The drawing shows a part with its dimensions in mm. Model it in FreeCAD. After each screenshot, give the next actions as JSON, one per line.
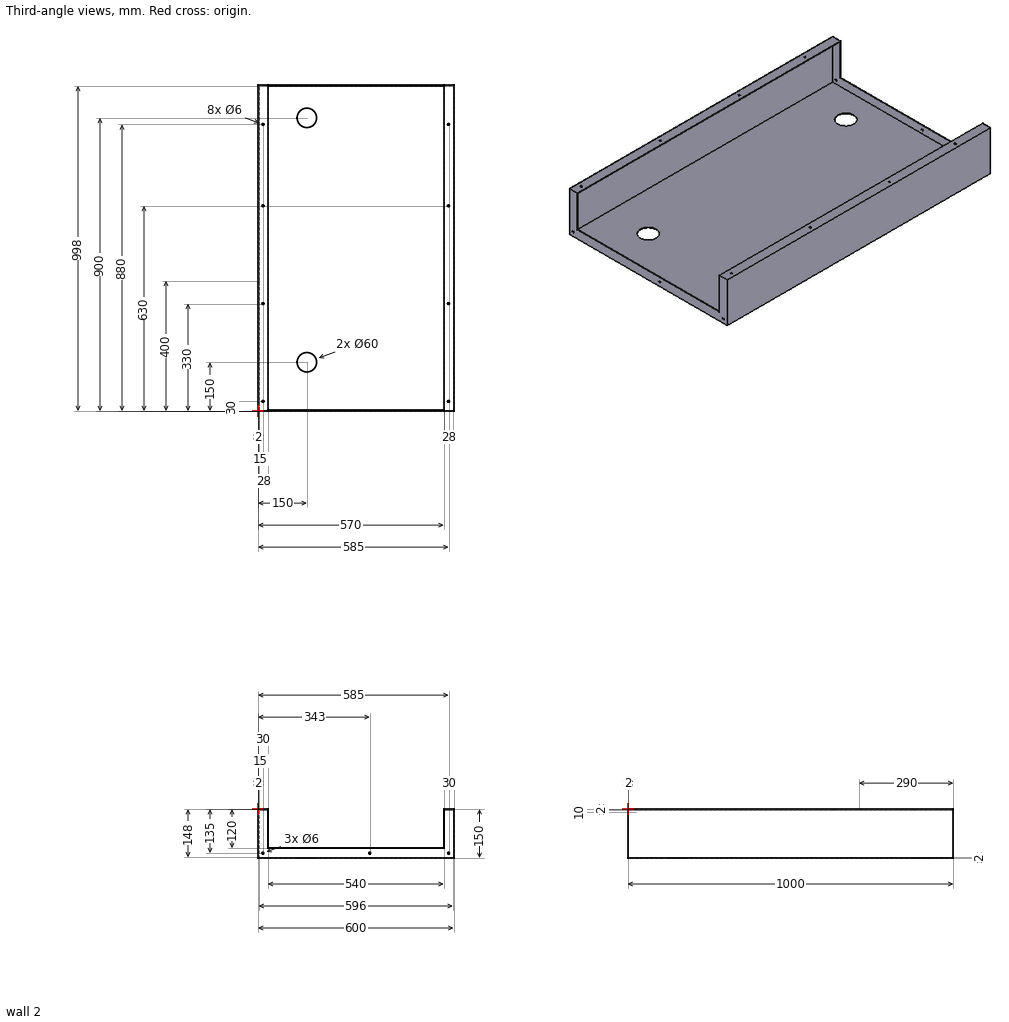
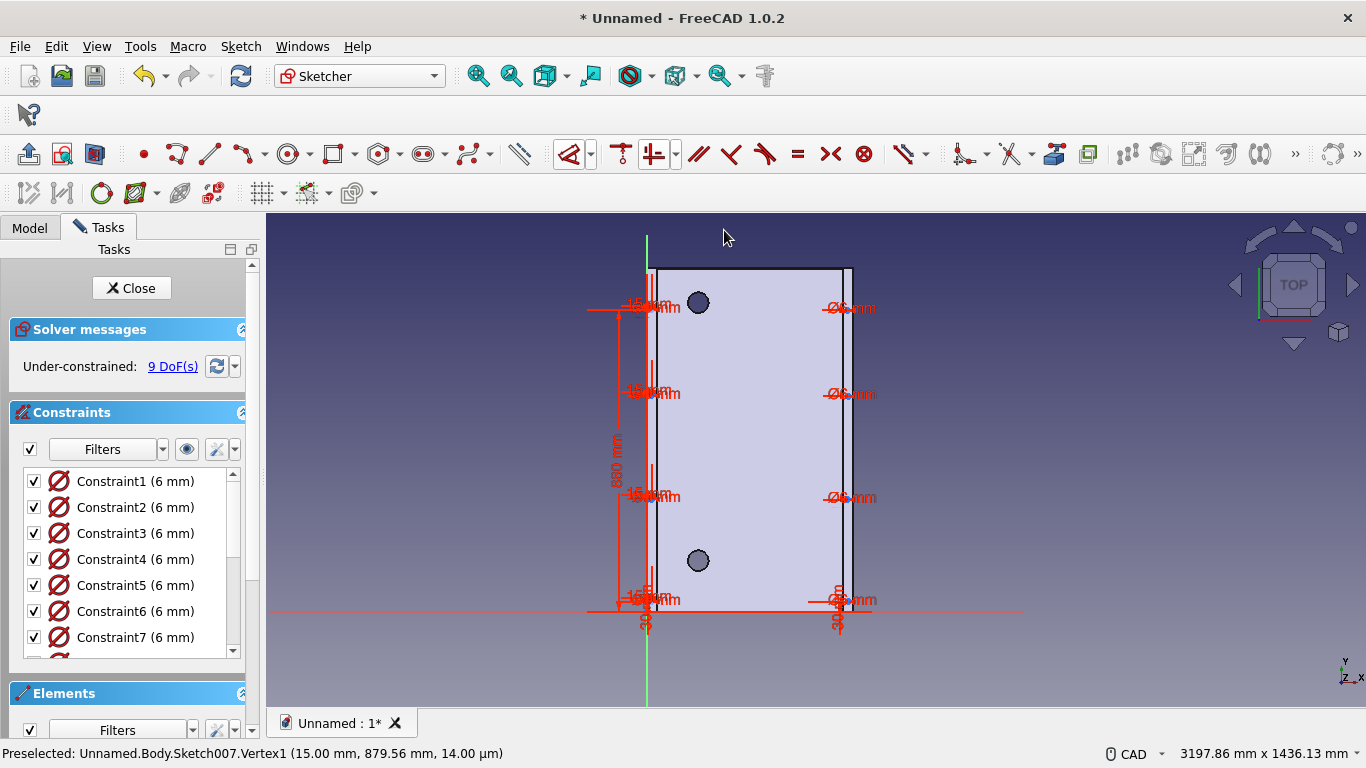
{"action": "left_click", "coordinate": [848, 310]}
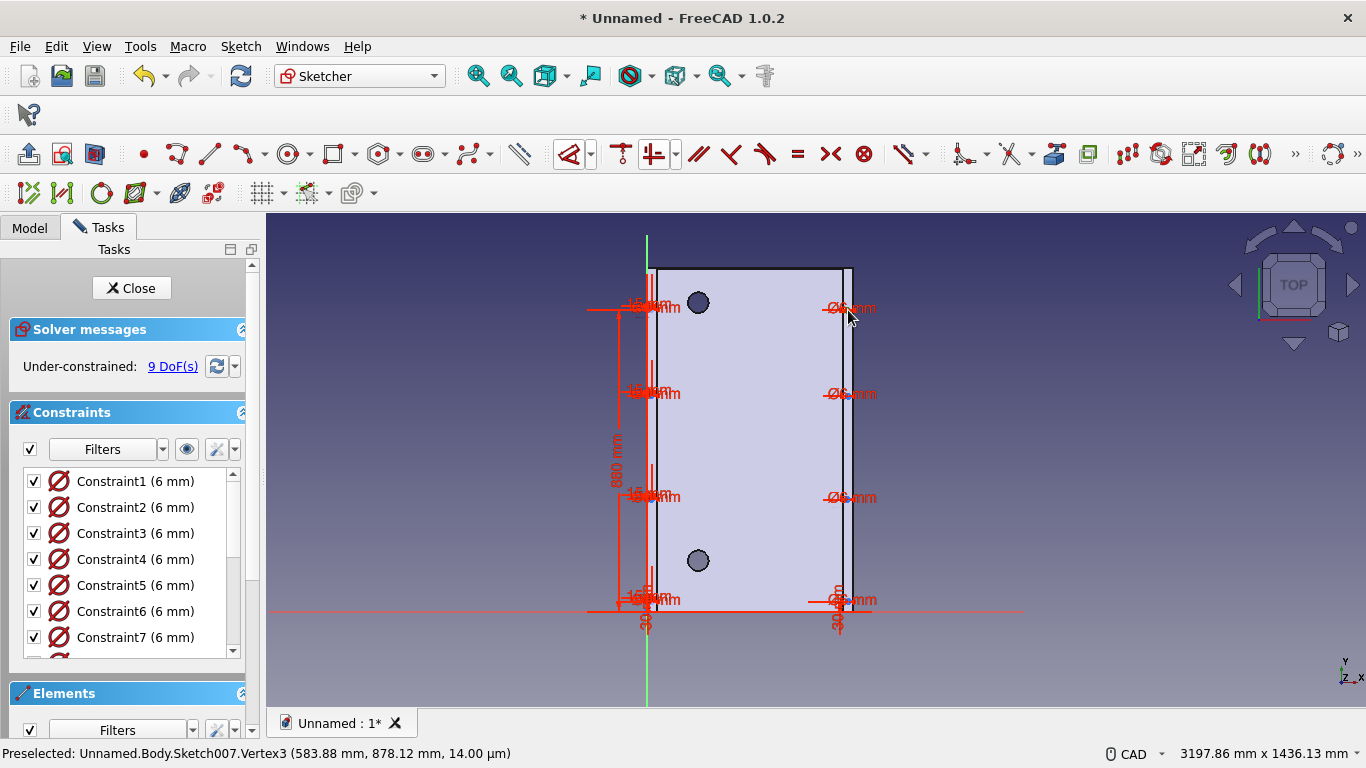
{"action": "left_click", "coordinate": [590, 154]}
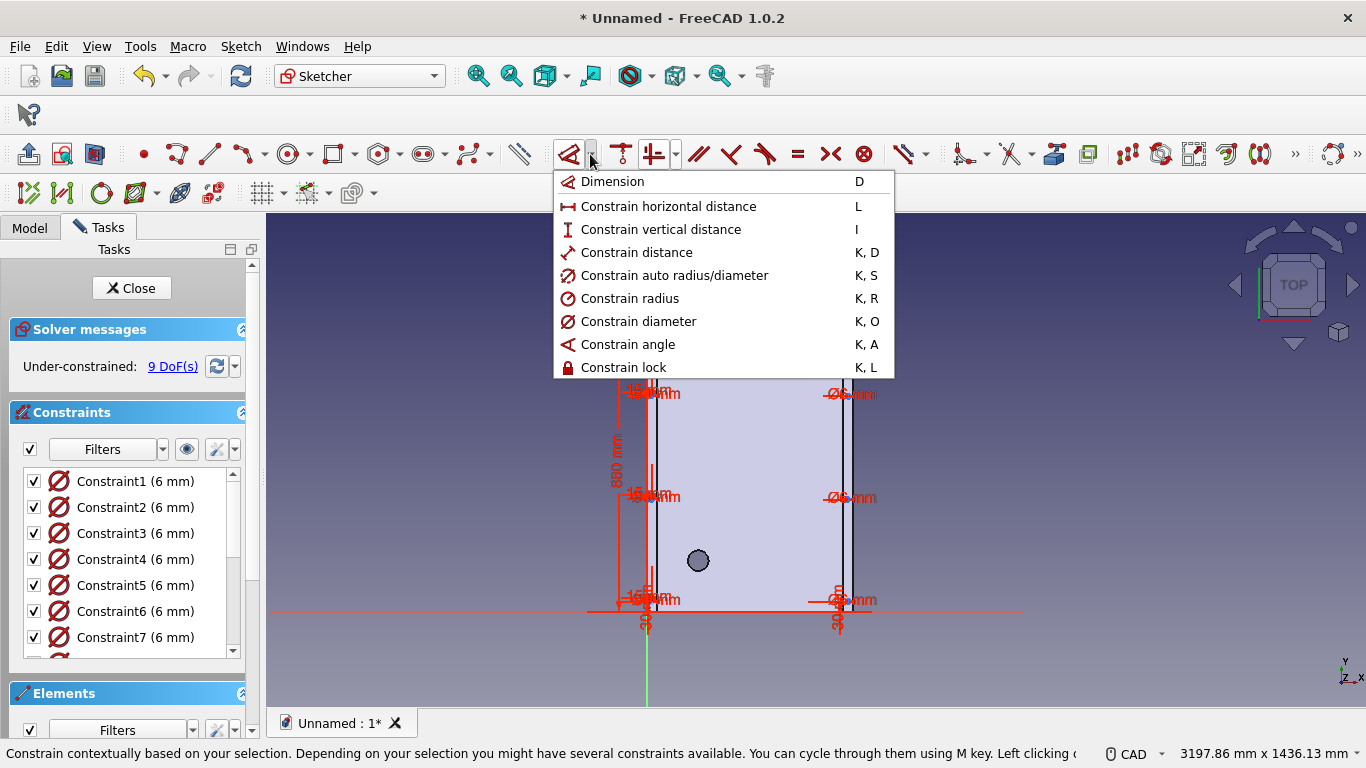
{"action": "left_click", "coordinate": [724, 206]}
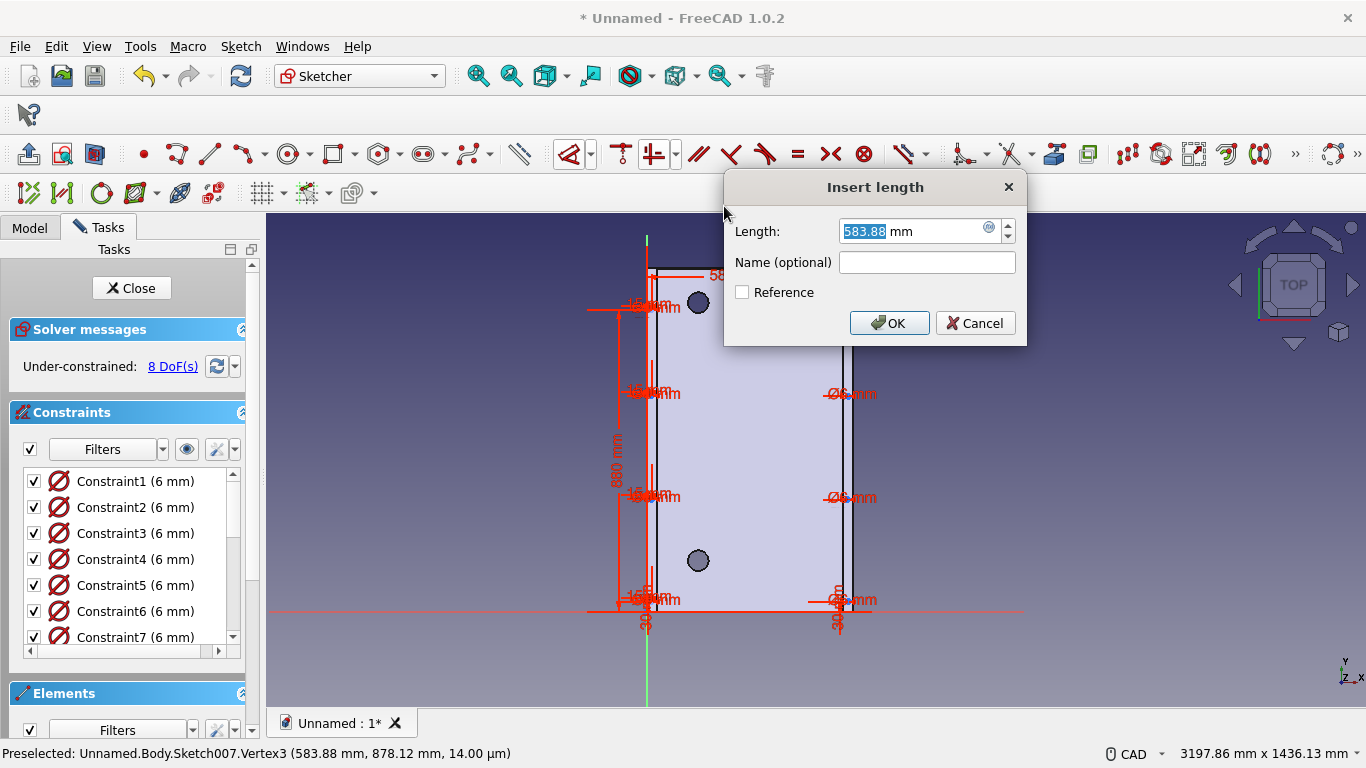
{"action": "type", "text": "585"}
{"action": "key", "text": "Return"}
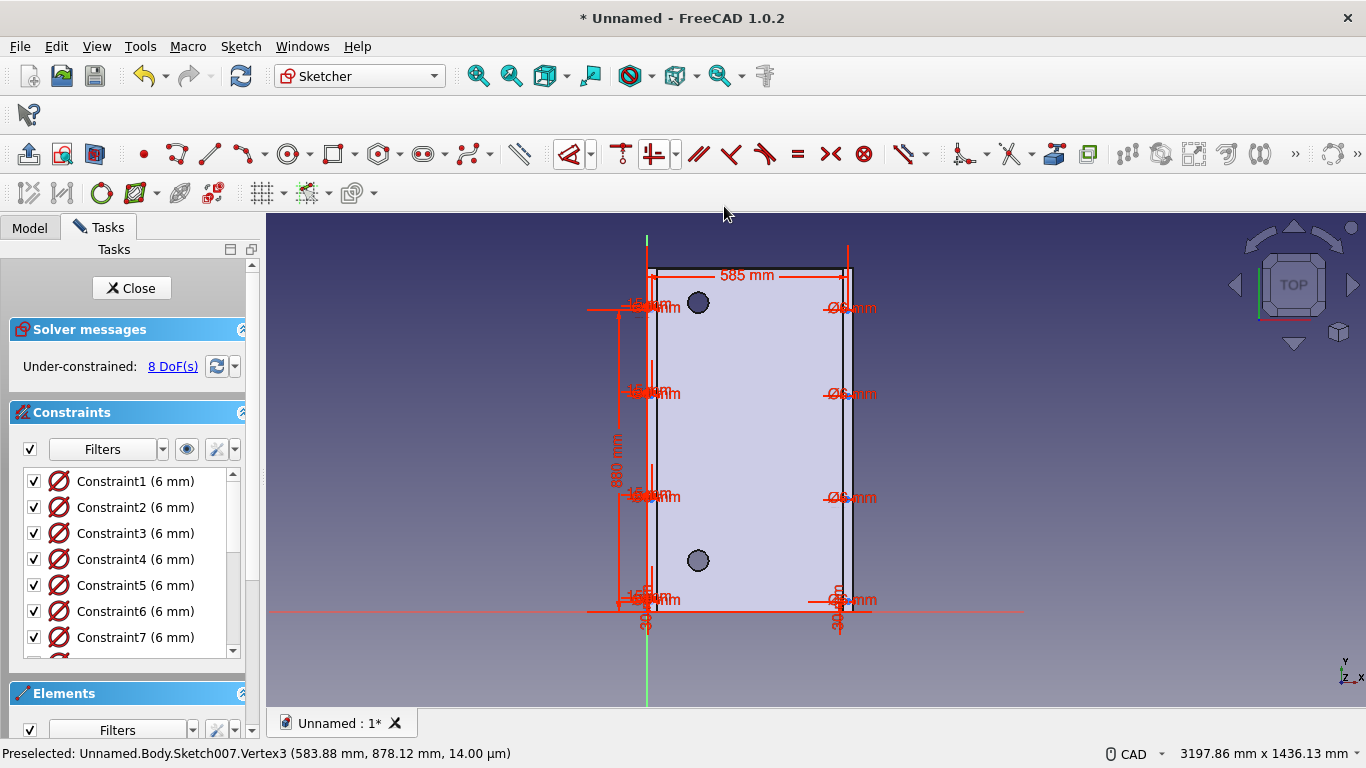
{"action": "left_click", "coordinate": [848, 310]}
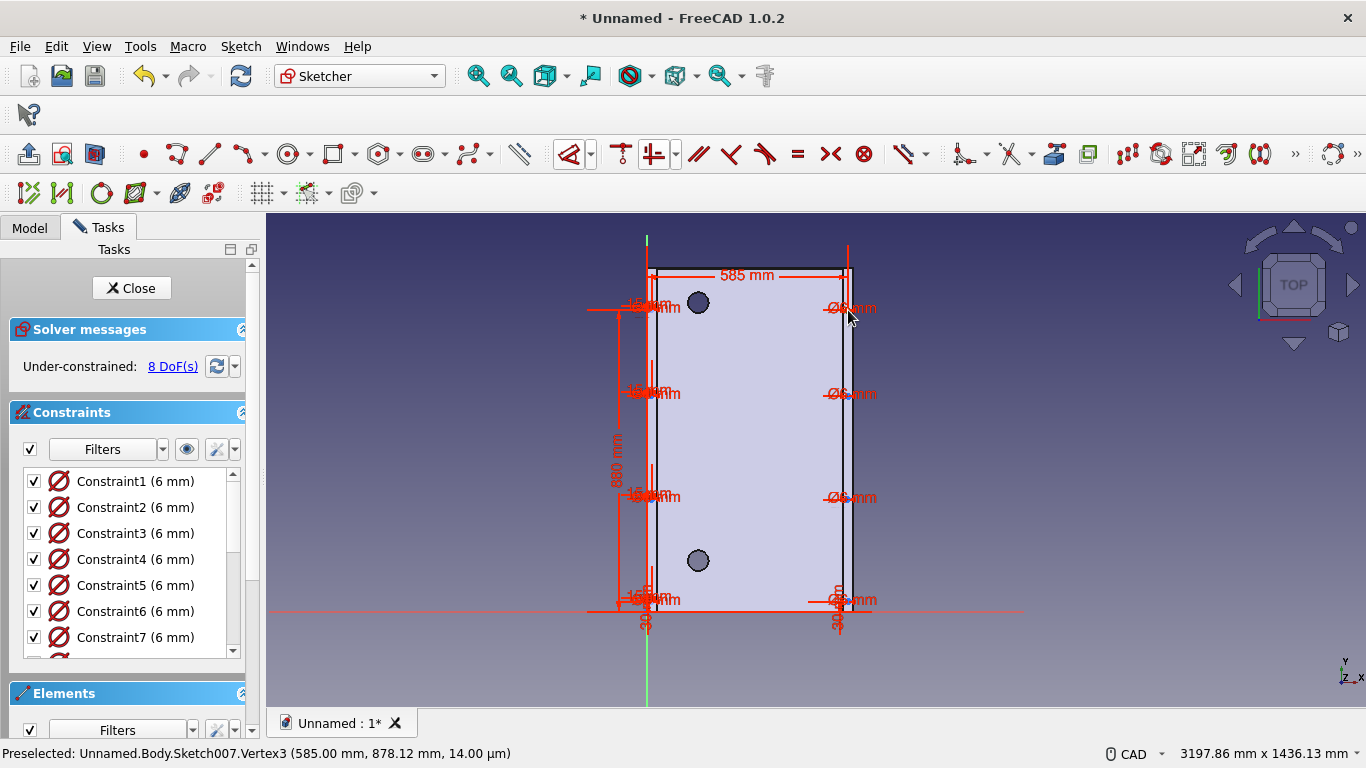
{"action": "left_click", "coordinate": [590, 154]}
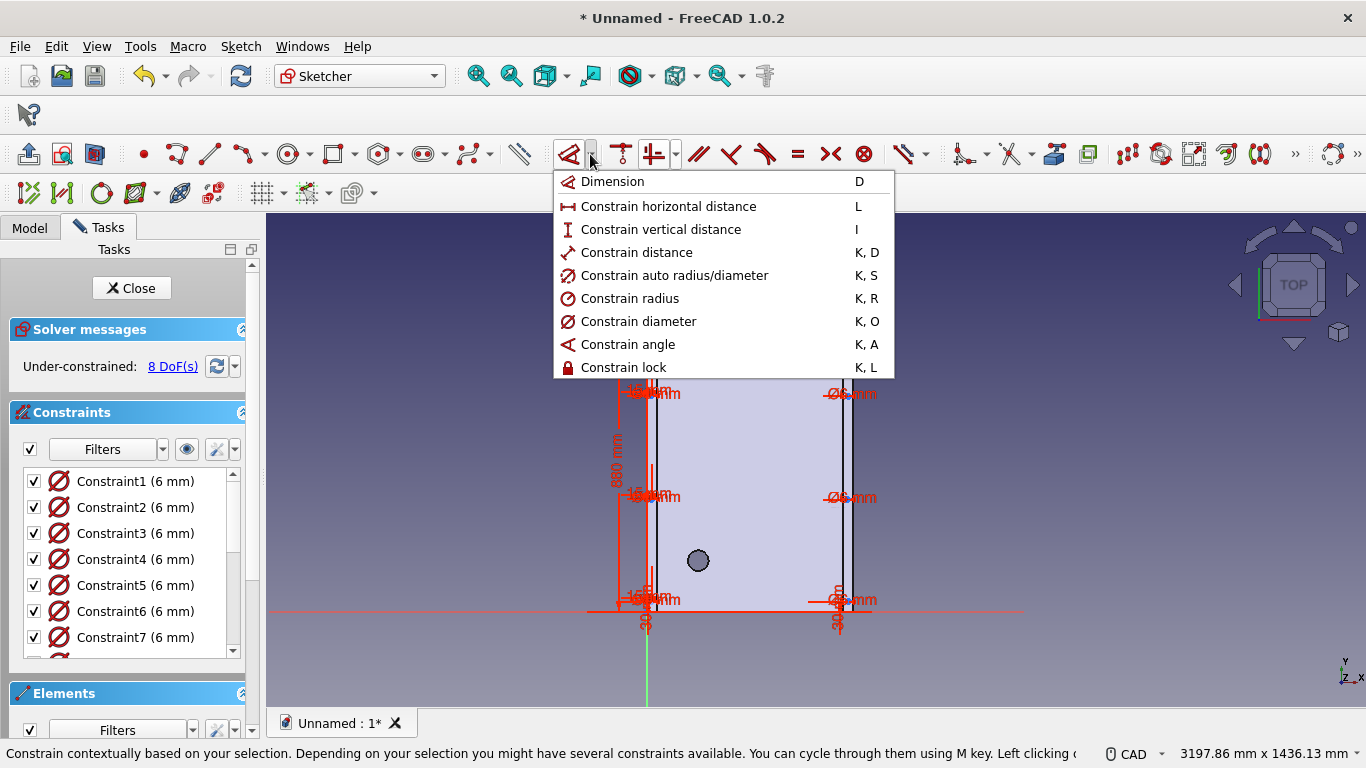
{"action": "left_click", "coordinate": [724, 230]}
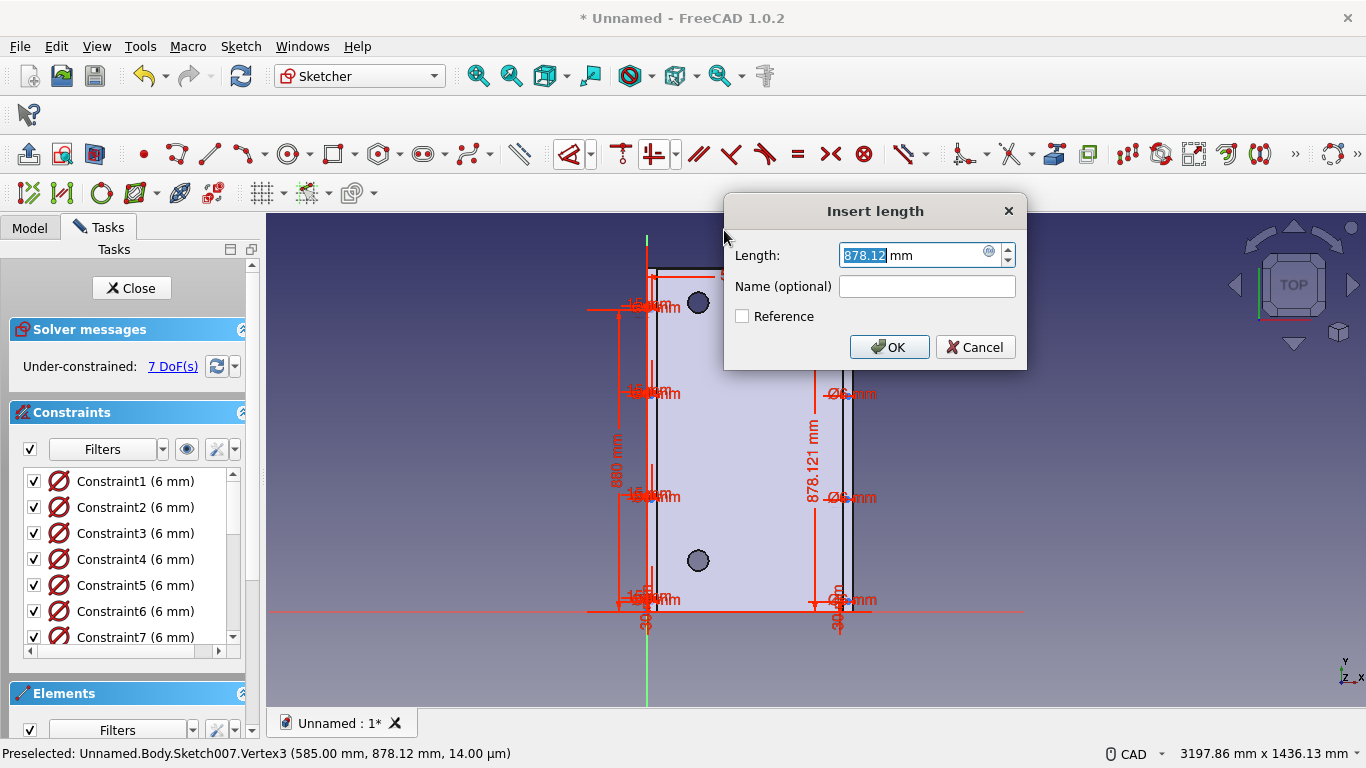
{"action": "type", "text": "880"}
{"action": "key", "text": "Return"}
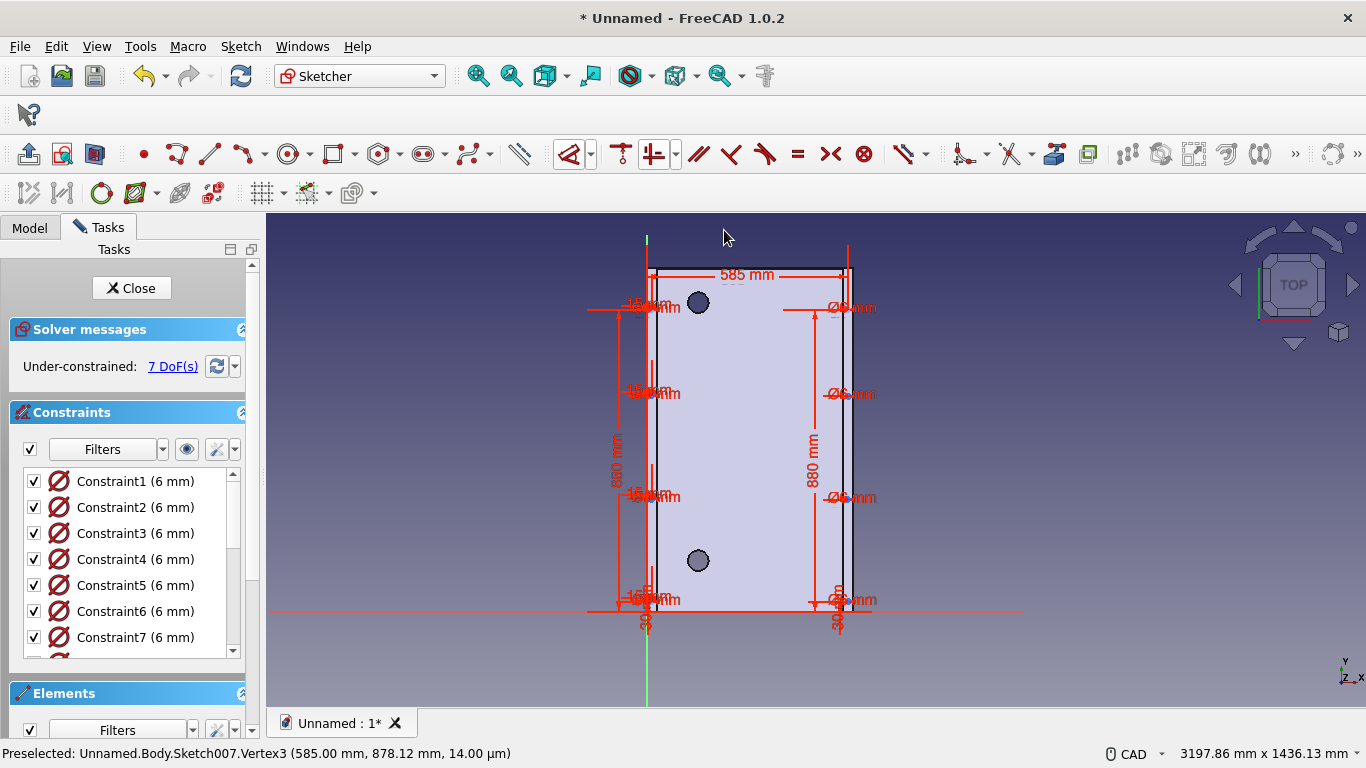
{"action": "left_click", "coordinate": [652, 499]}